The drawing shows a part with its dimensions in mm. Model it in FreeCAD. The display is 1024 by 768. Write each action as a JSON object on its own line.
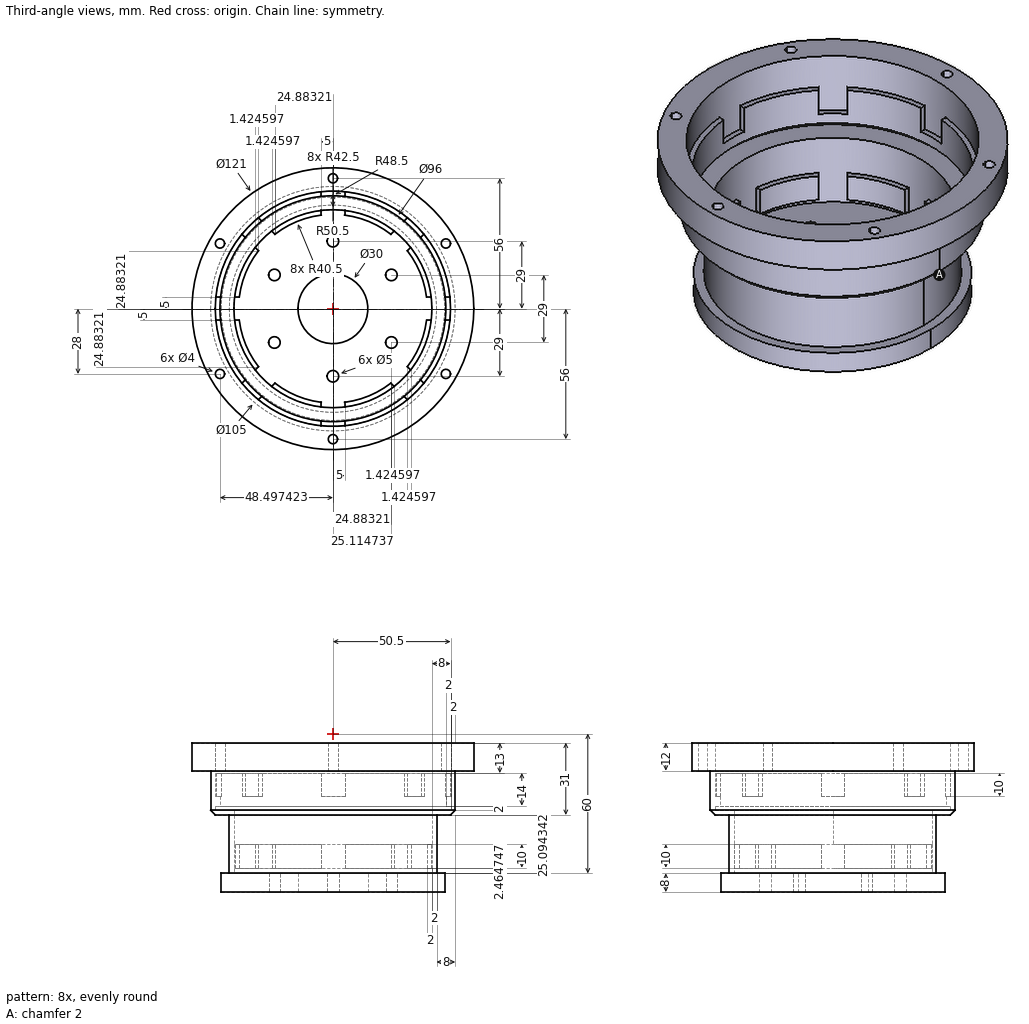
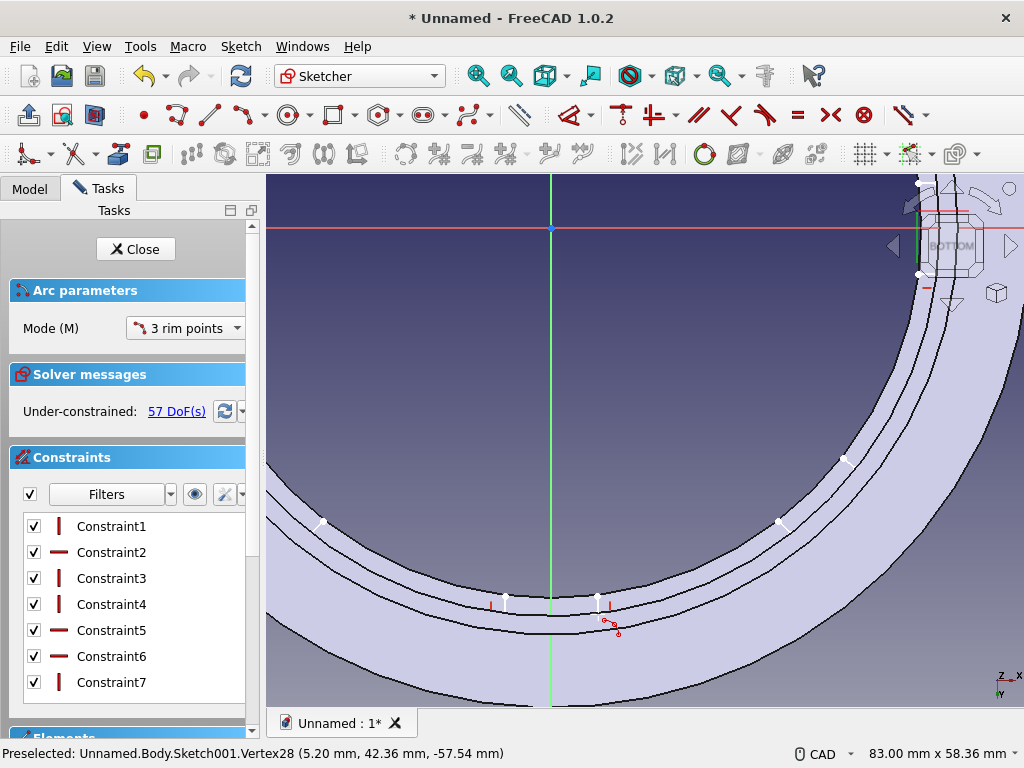
{"action": "scroll", "coordinate": [506, 595], "scroll_direction": "up", "scroll_amount": 3}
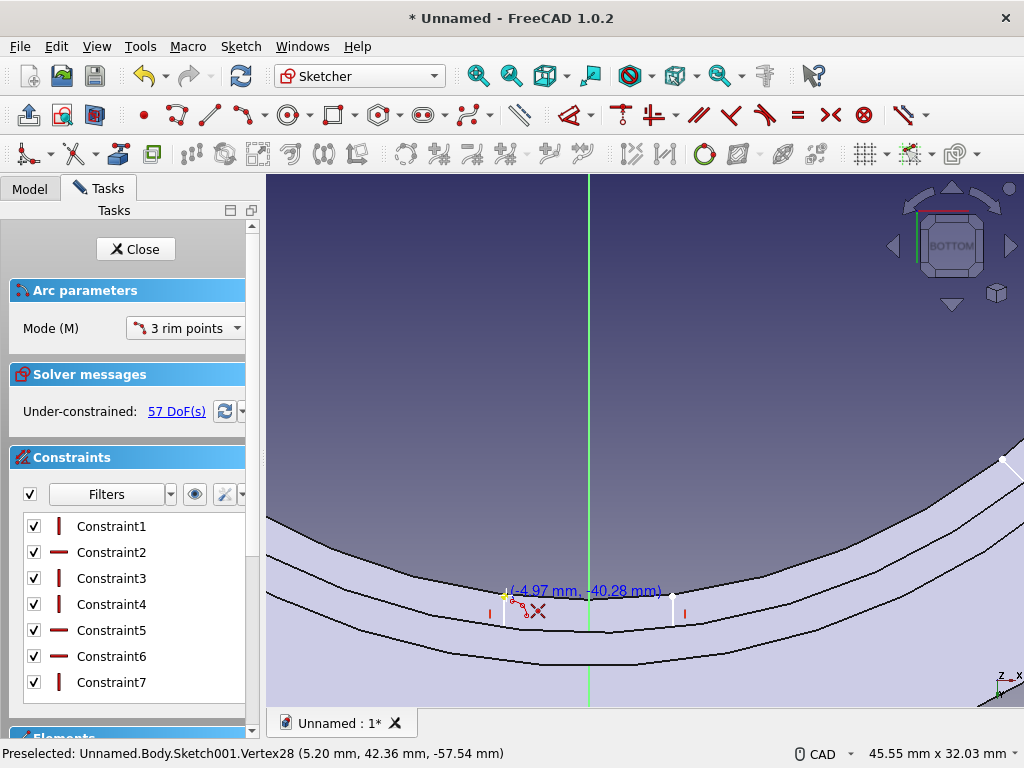
{"action": "left_click", "coordinate": [504, 596]}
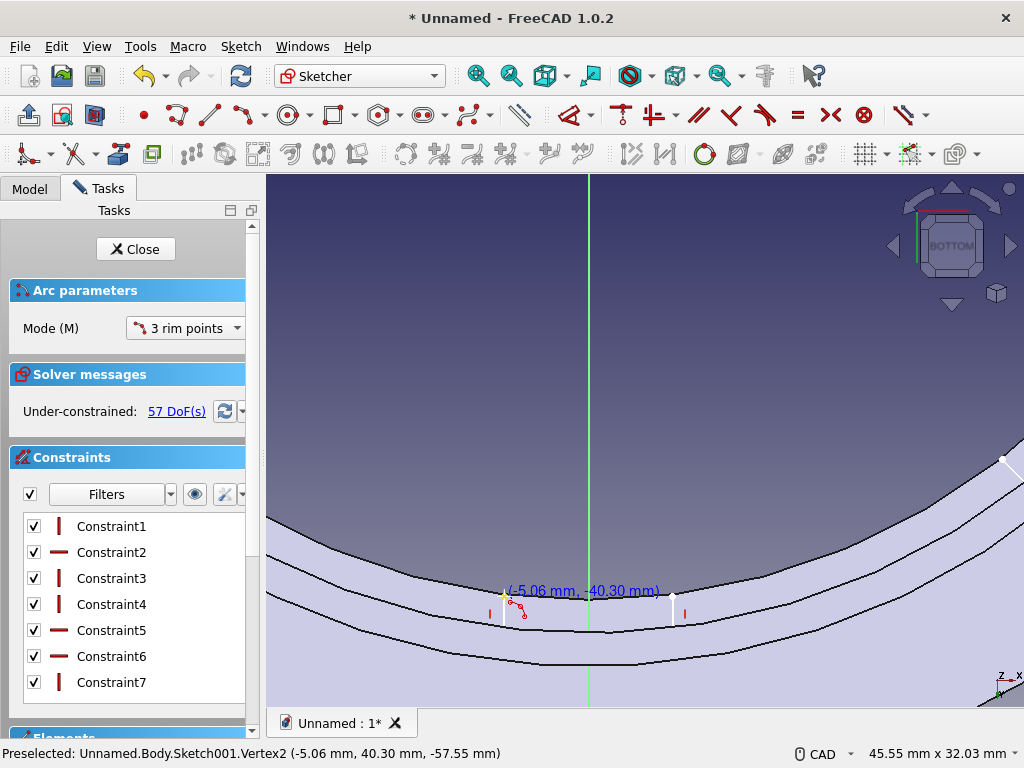
{"action": "scroll", "coordinate": [573, 609], "scroll_direction": "down", "scroll_amount": 7}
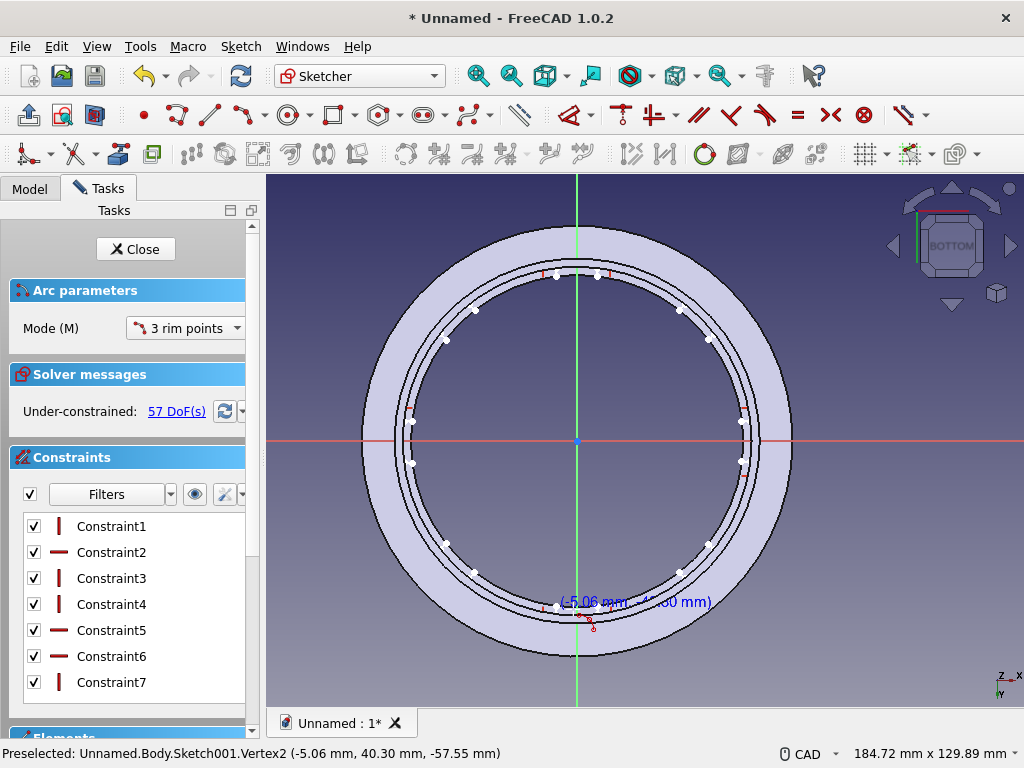
{"action": "scroll", "coordinate": [475, 572], "scroll_direction": "up", "scroll_amount": 7}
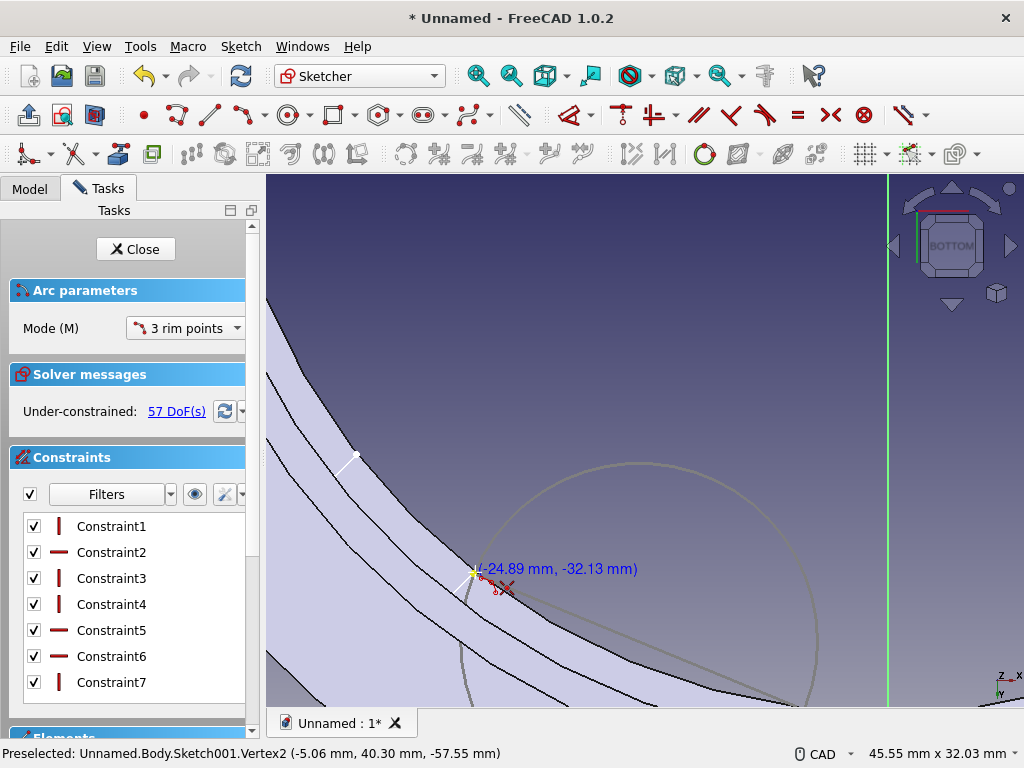
{"action": "left_click", "coordinate": [473, 573]}
{"action": "left_click", "coordinate": [630, 662]}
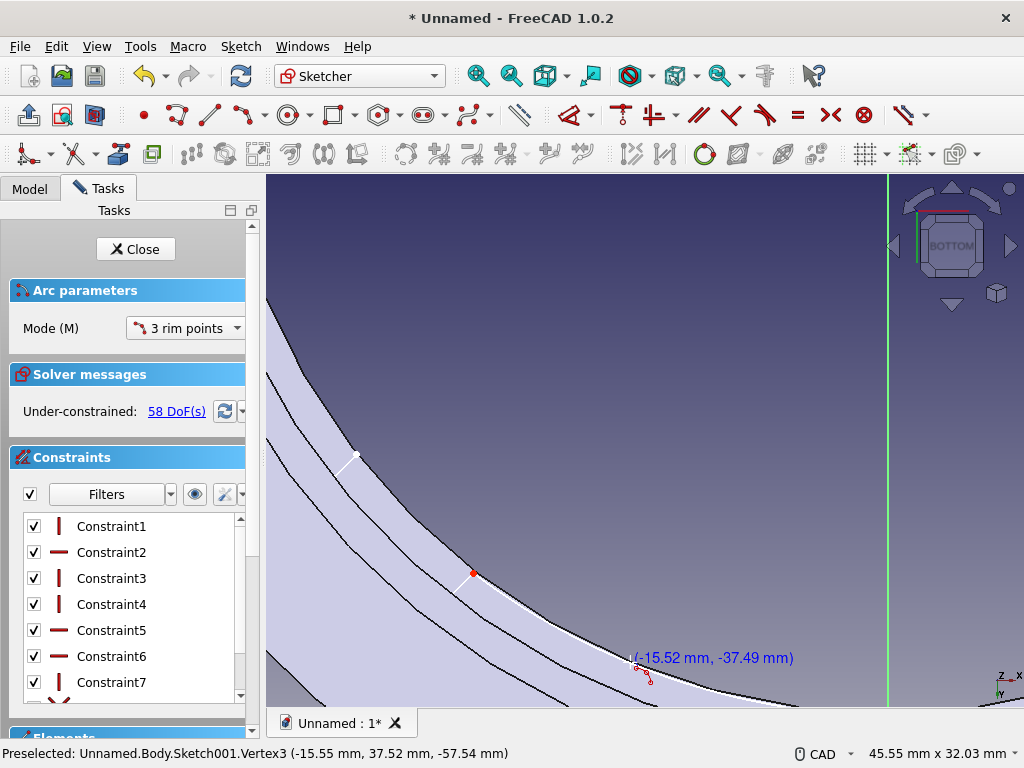
{"action": "left_click", "coordinate": [450, 597]}
{"action": "left_click", "coordinate": [333, 478]}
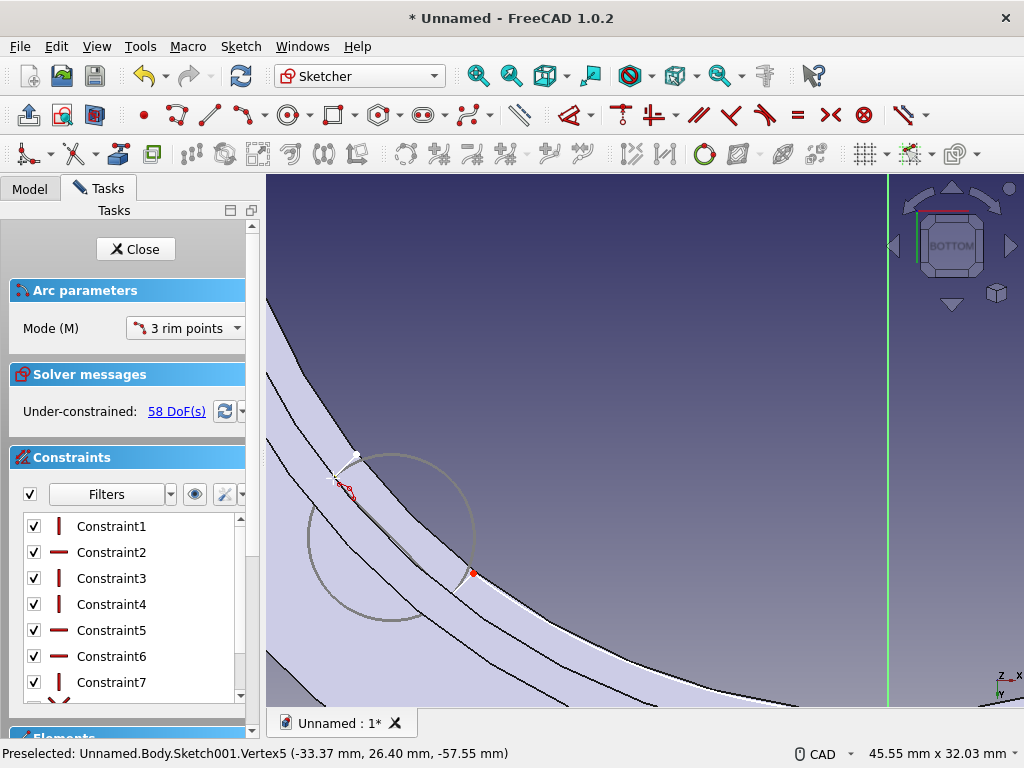
{"action": "scroll", "coordinate": [388, 539], "scroll_direction": "up", "scroll_amount": 6}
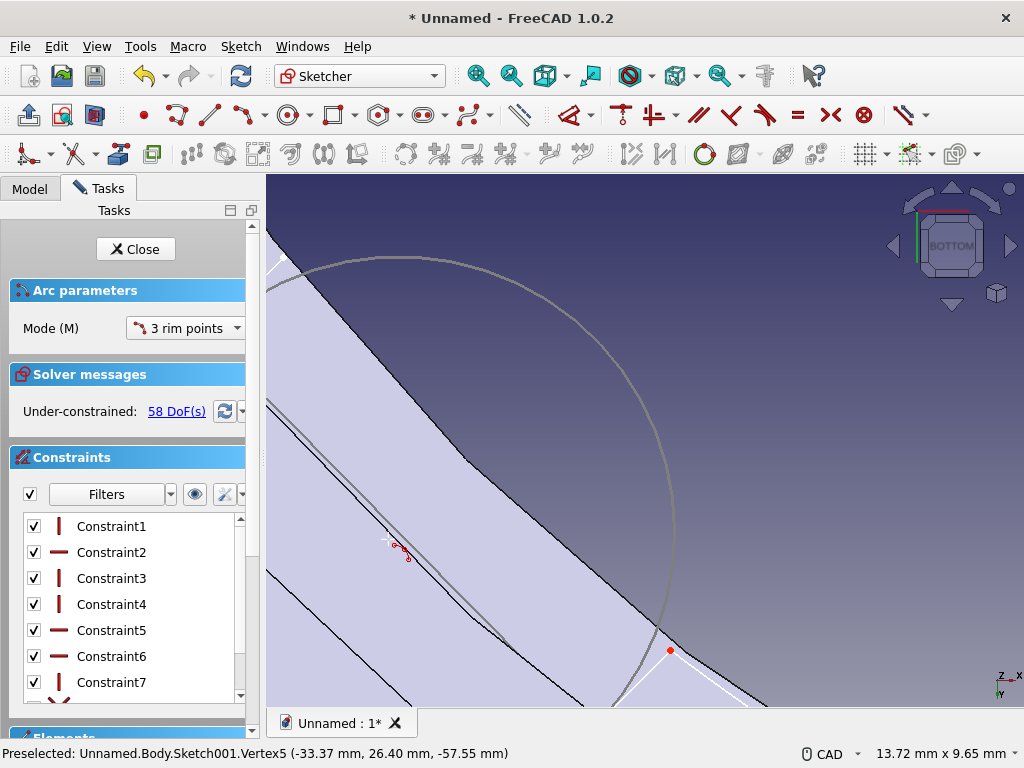
{"action": "left_click", "coordinate": [388, 538]}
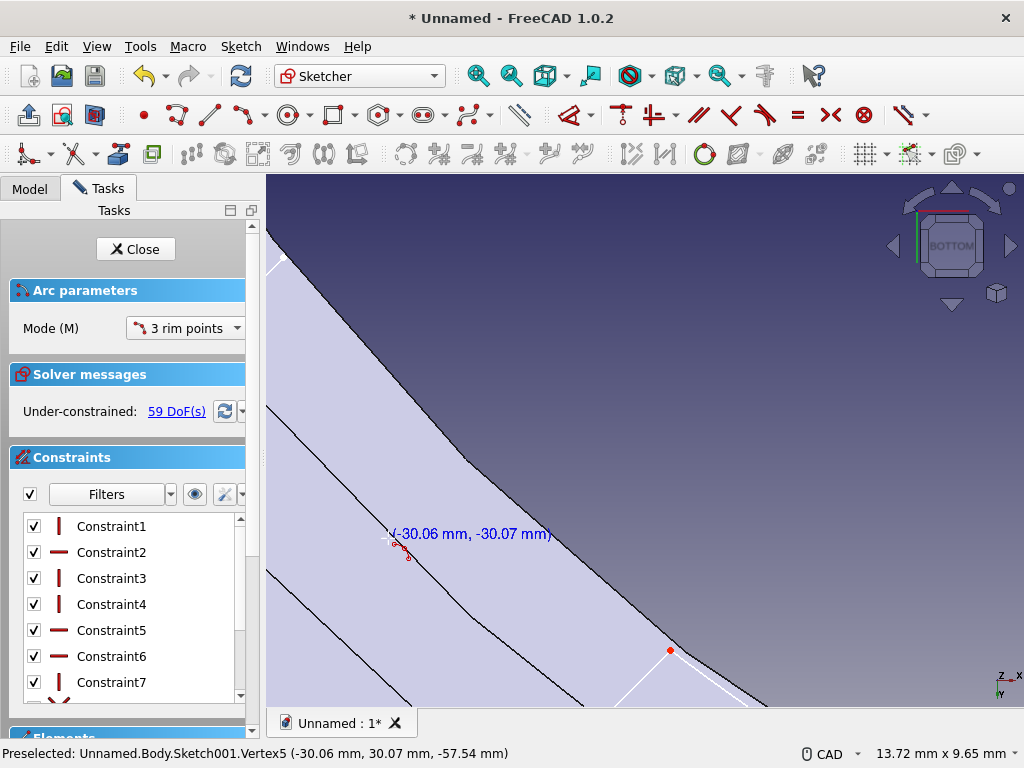
{"action": "scroll", "coordinate": [458, 566], "scroll_direction": "down", "scroll_amount": 13}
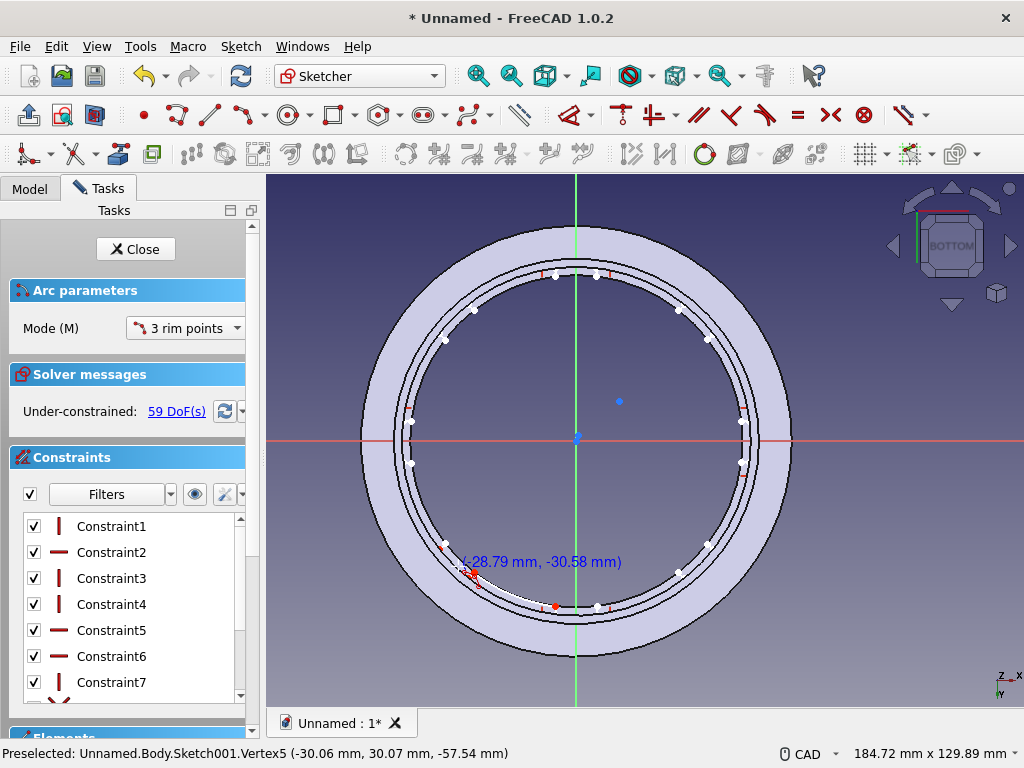
{"action": "scroll", "coordinate": [445, 543], "scroll_direction": "up", "scroll_amount": 7}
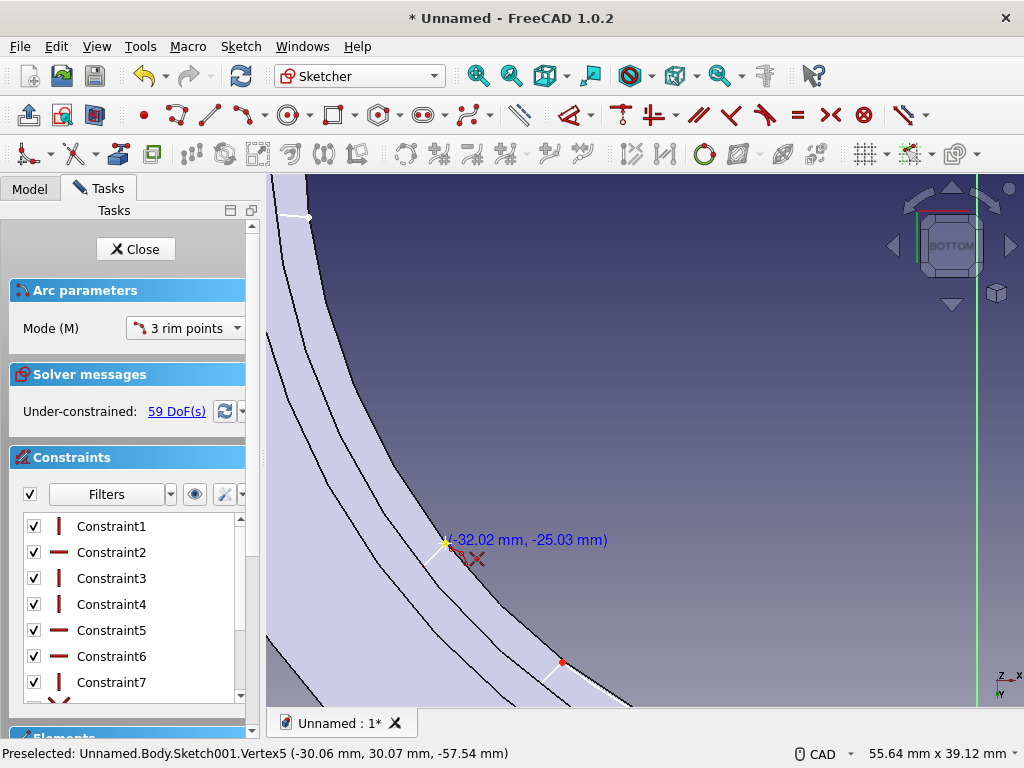
{"action": "left_click", "coordinate": [445, 544]}
{"action": "left_click", "coordinate": [309, 217]}
{"action": "left_click", "coordinate": [354, 386]}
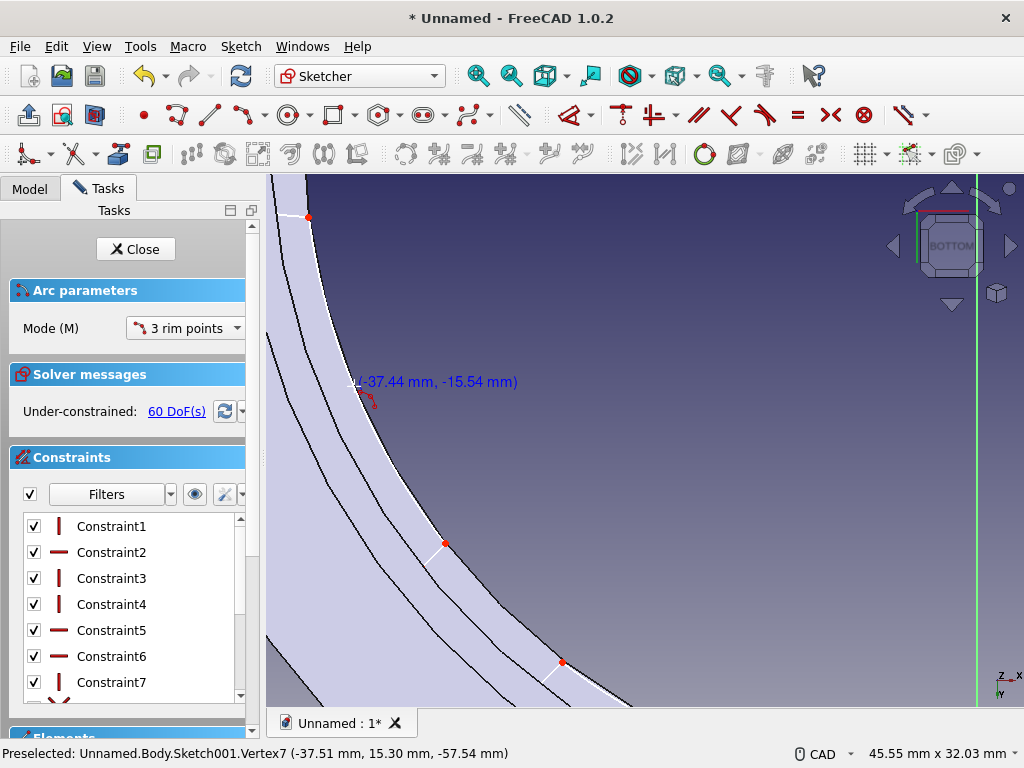
{"action": "scroll", "coordinate": [445, 543], "scroll_direction": "down", "scroll_amount": 7}